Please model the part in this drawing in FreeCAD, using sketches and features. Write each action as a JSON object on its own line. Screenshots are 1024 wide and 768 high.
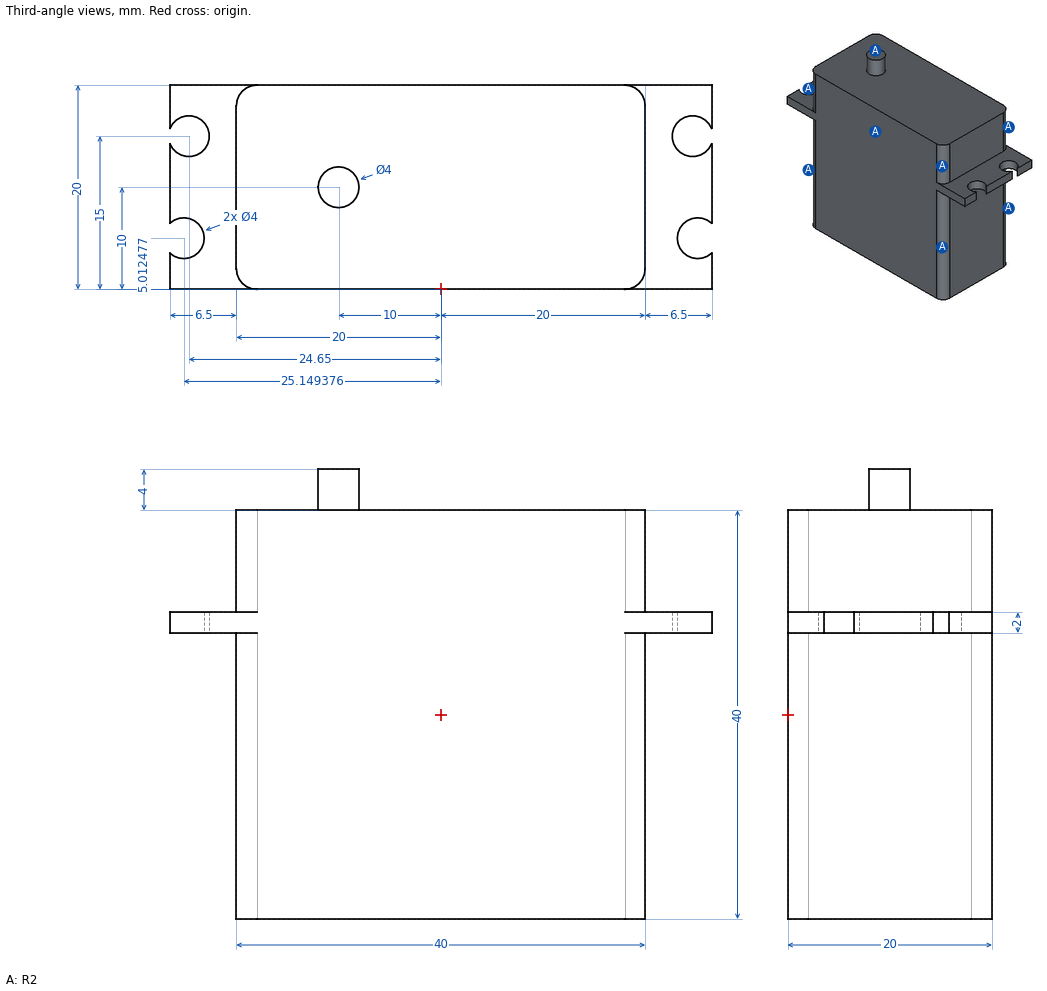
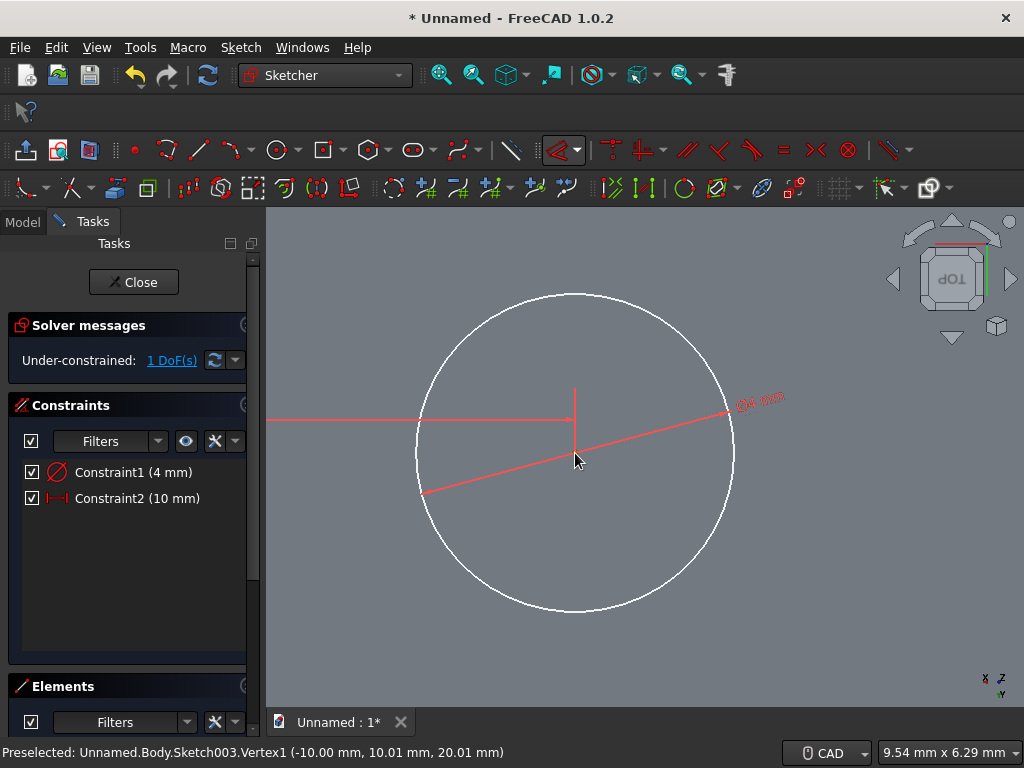
{"action": "key", "text": "i"}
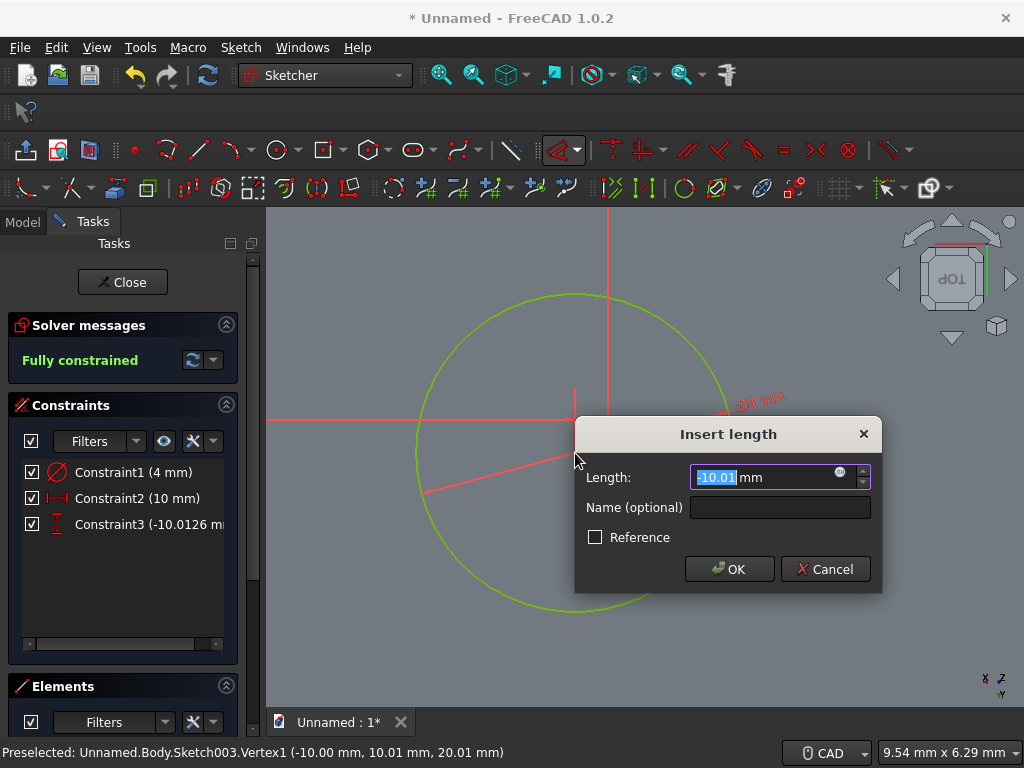
{"action": "type", "text": "-10"}
{"action": "key", "text": "Return"}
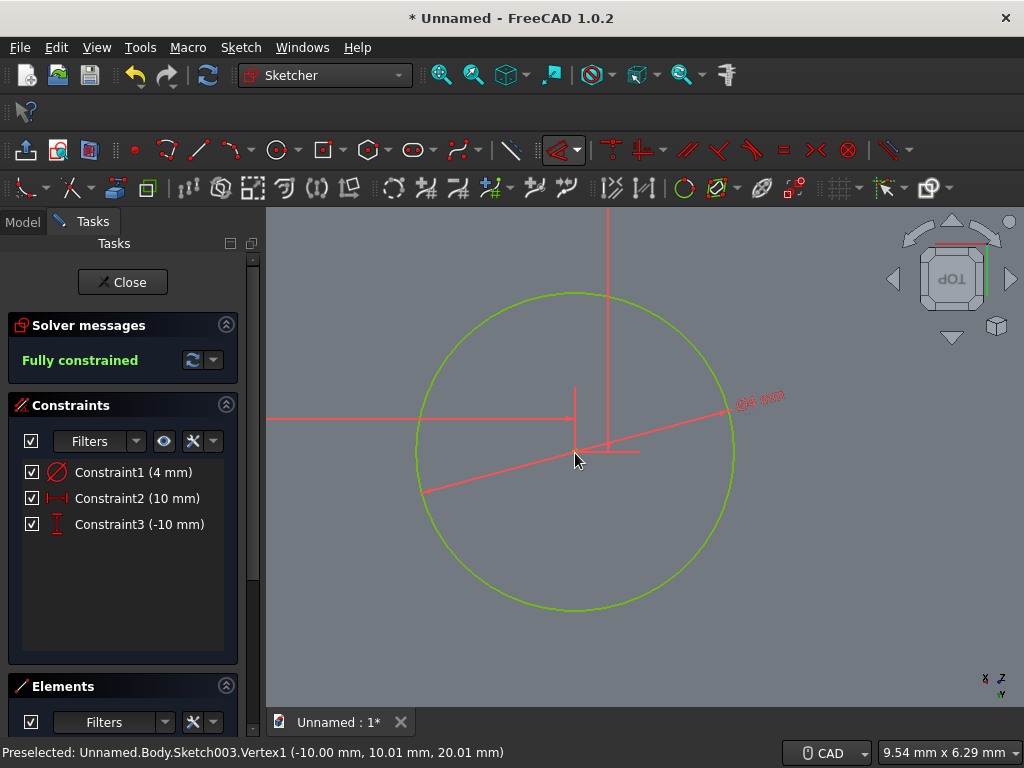
{"action": "left_click", "coordinate": [123, 282]}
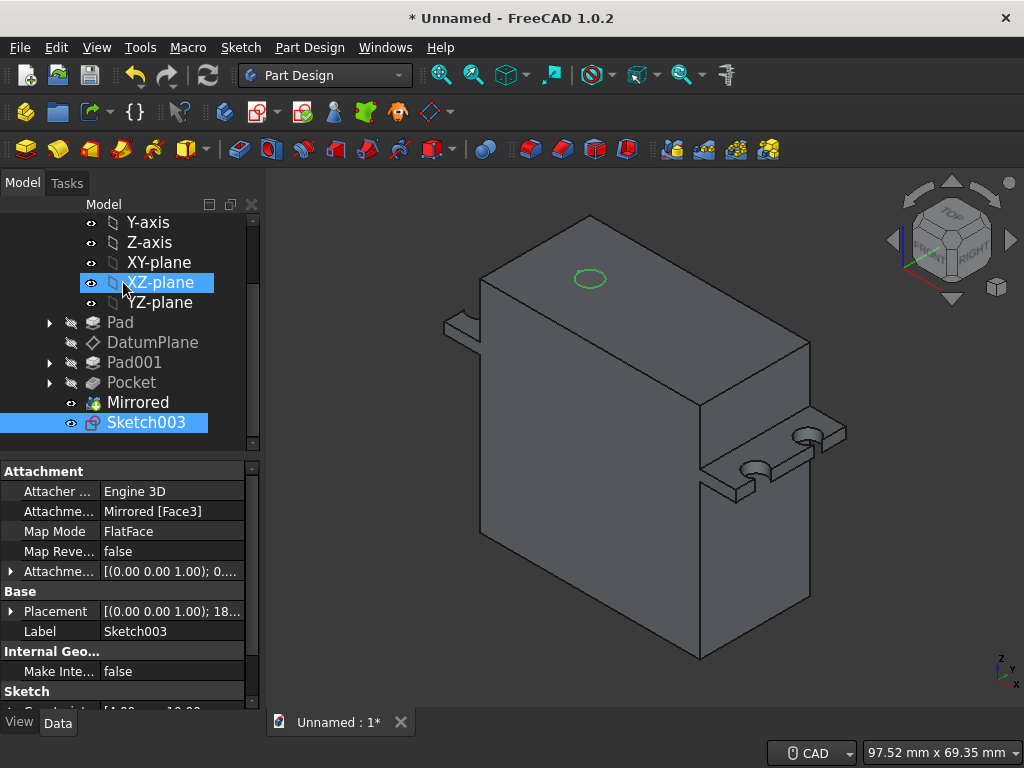
{"action": "left_click", "coordinate": [26, 150]}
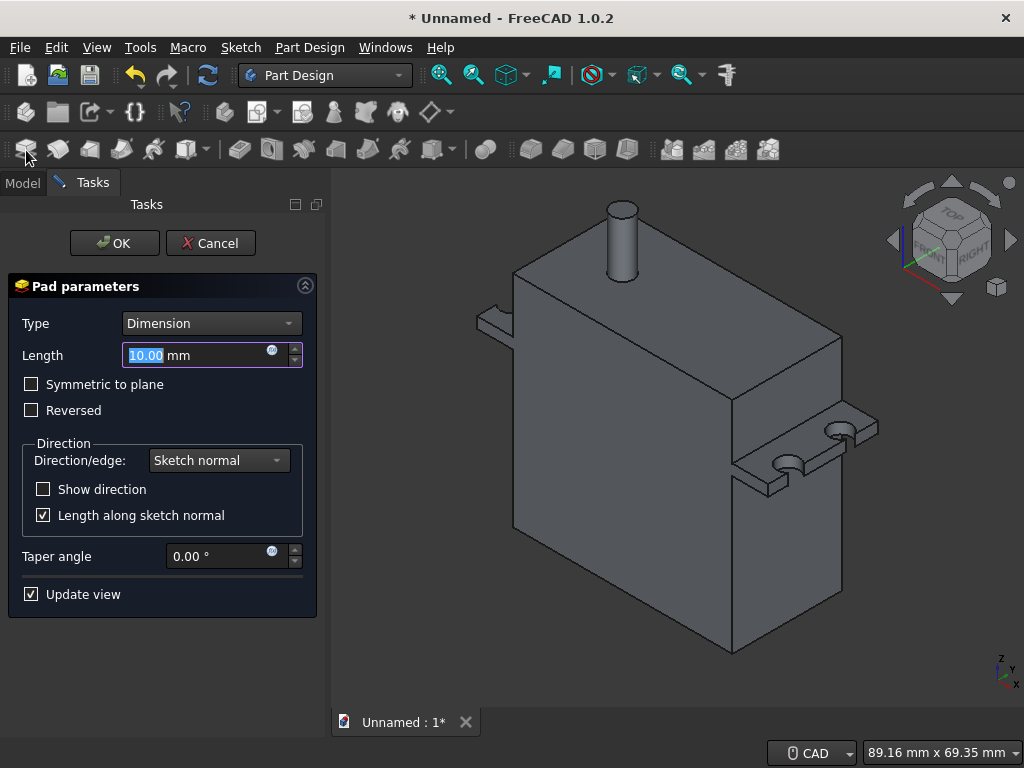
{"action": "type", "text": "4"}
{"action": "key", "text": "Tab"}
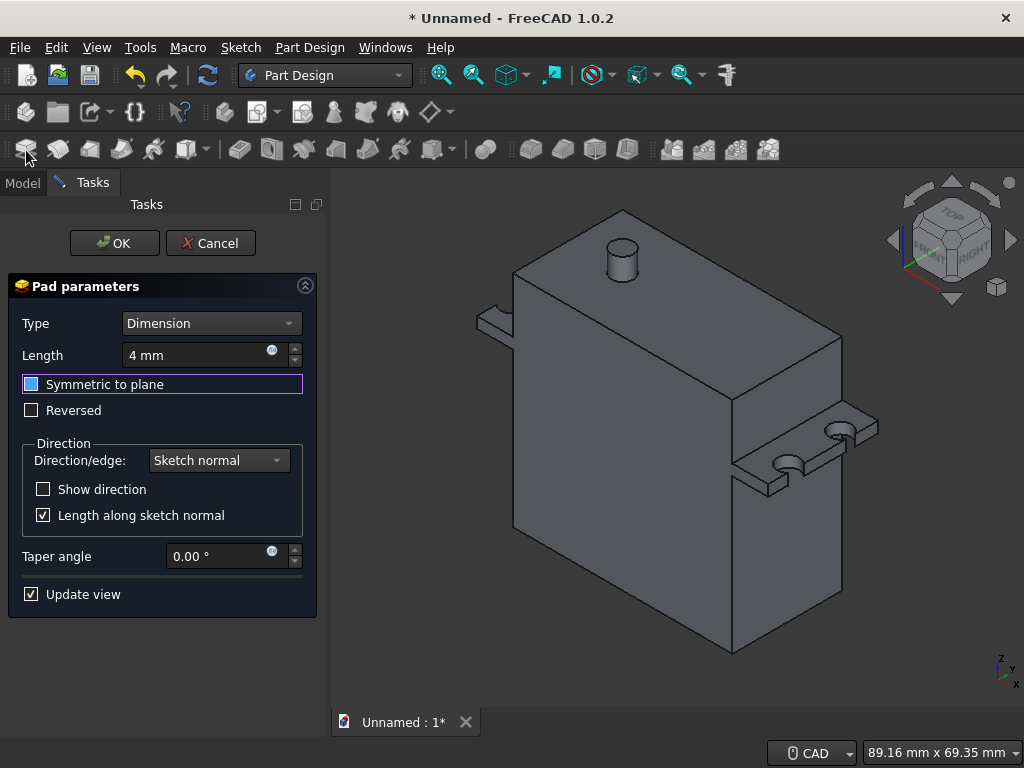
{"action": "left_click", "coordinate": [115, 243]}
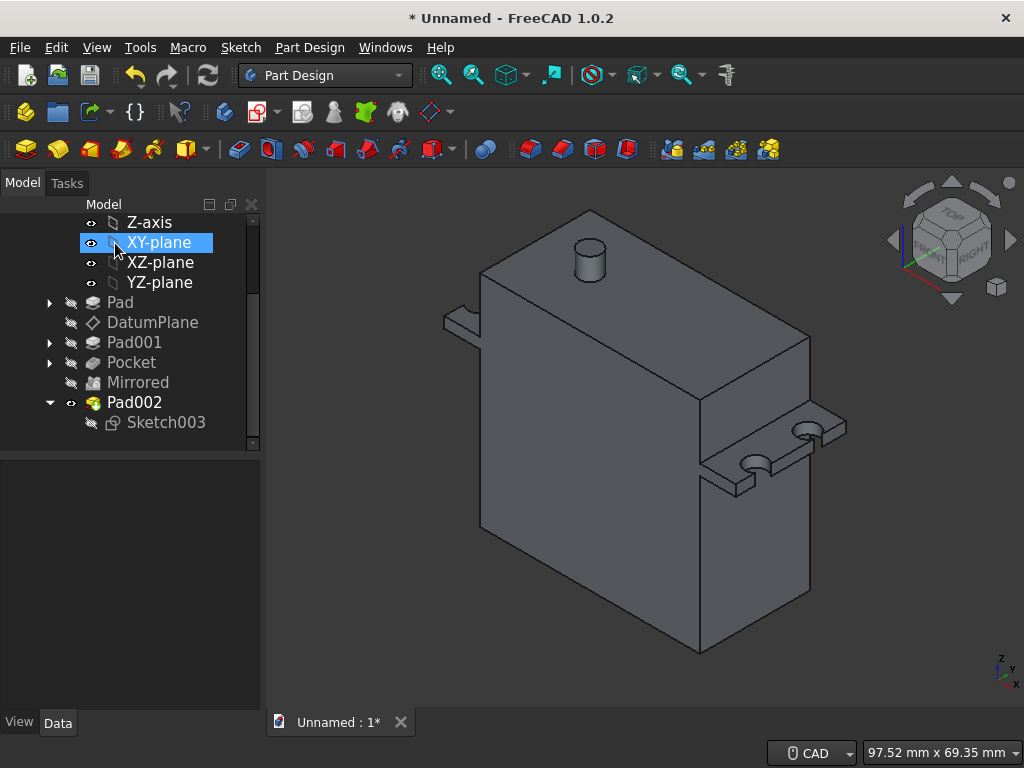
{"action": "key", "text": "v f"}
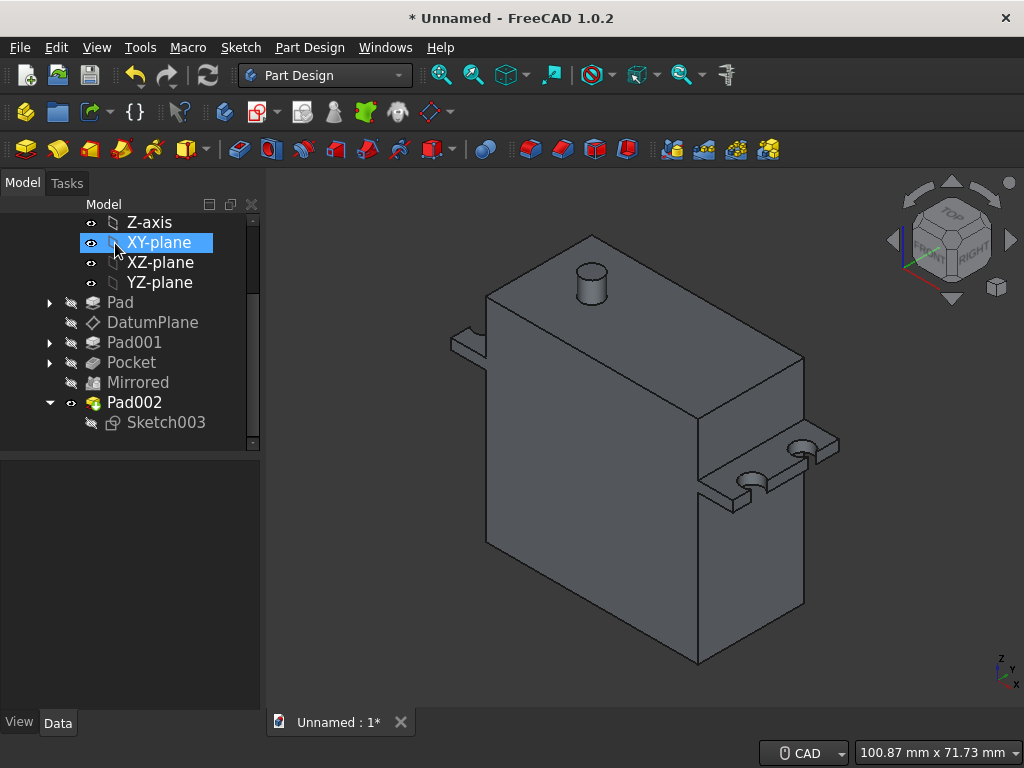
{"action": "left_click", "coordinate": [698, 578]}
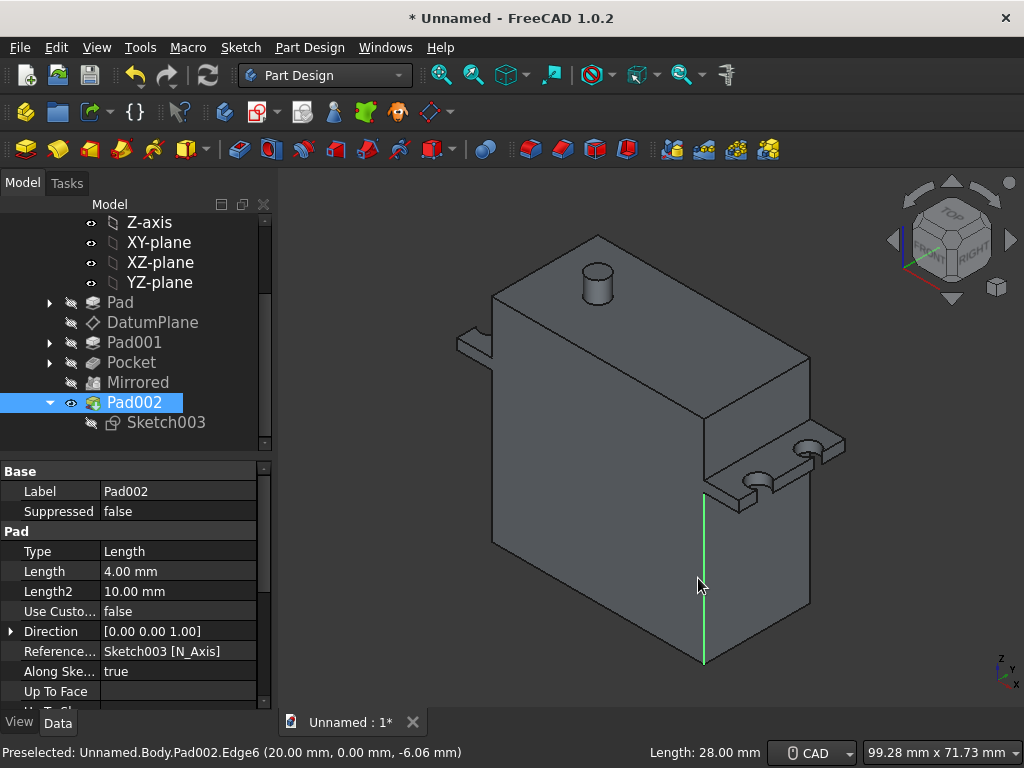
{"action": "left_click", "coordinate": [704, 449], "text": "ctrl"}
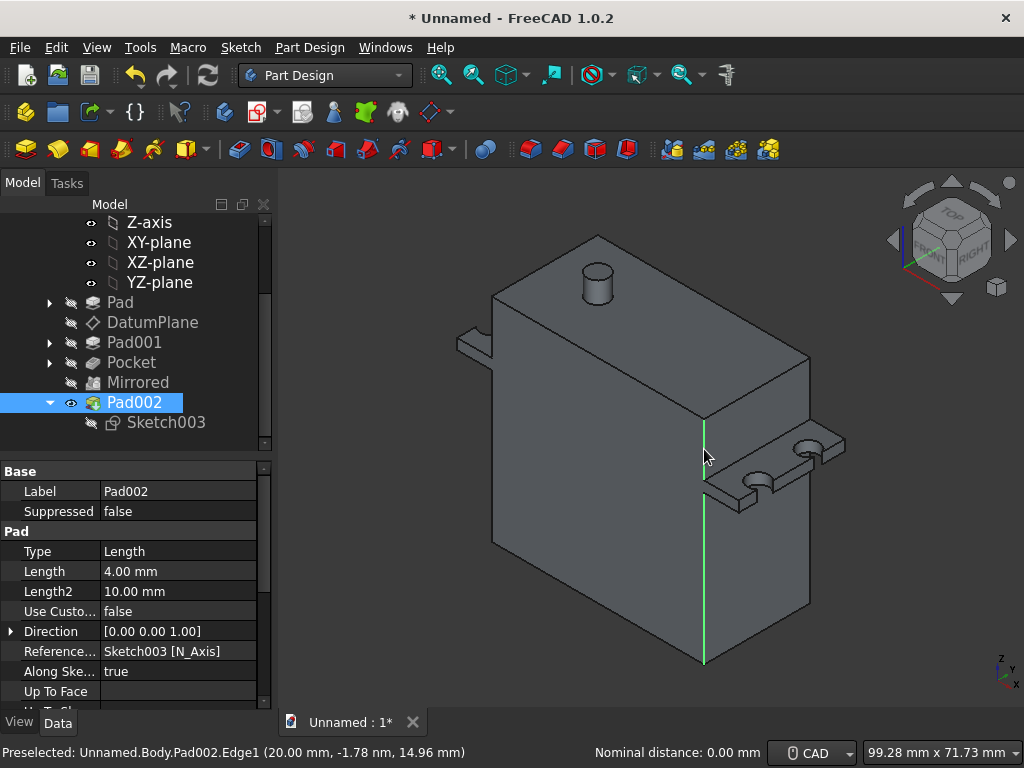
{"action": "key", "text": "2"}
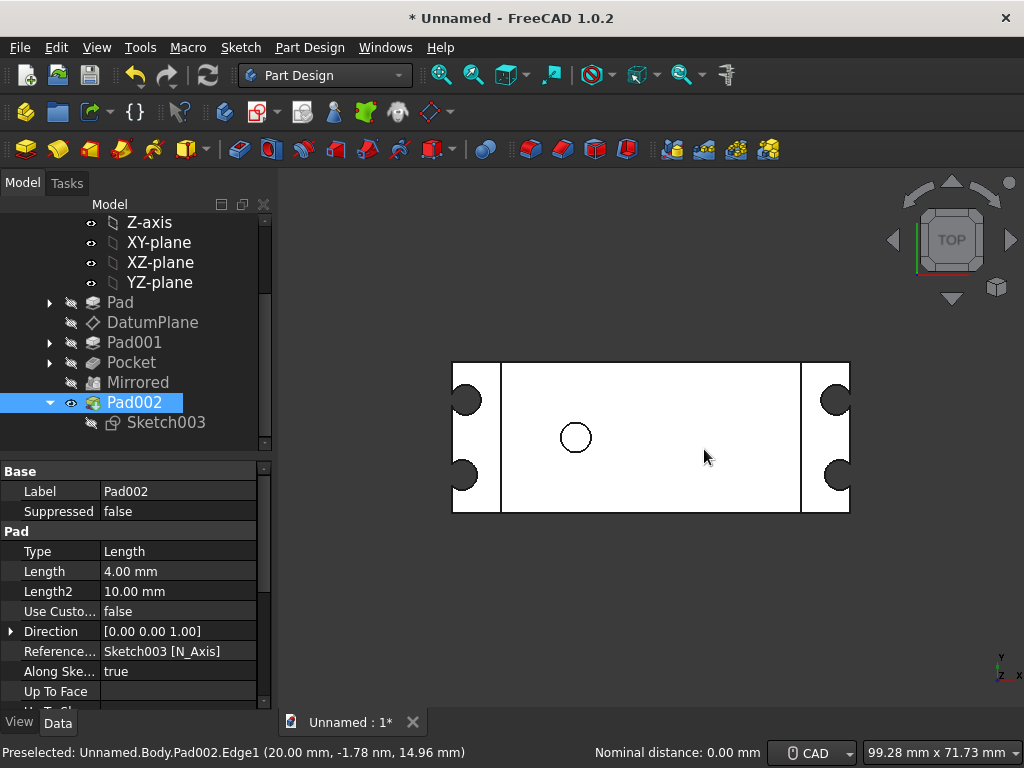
{"action": "key", "text": "0"}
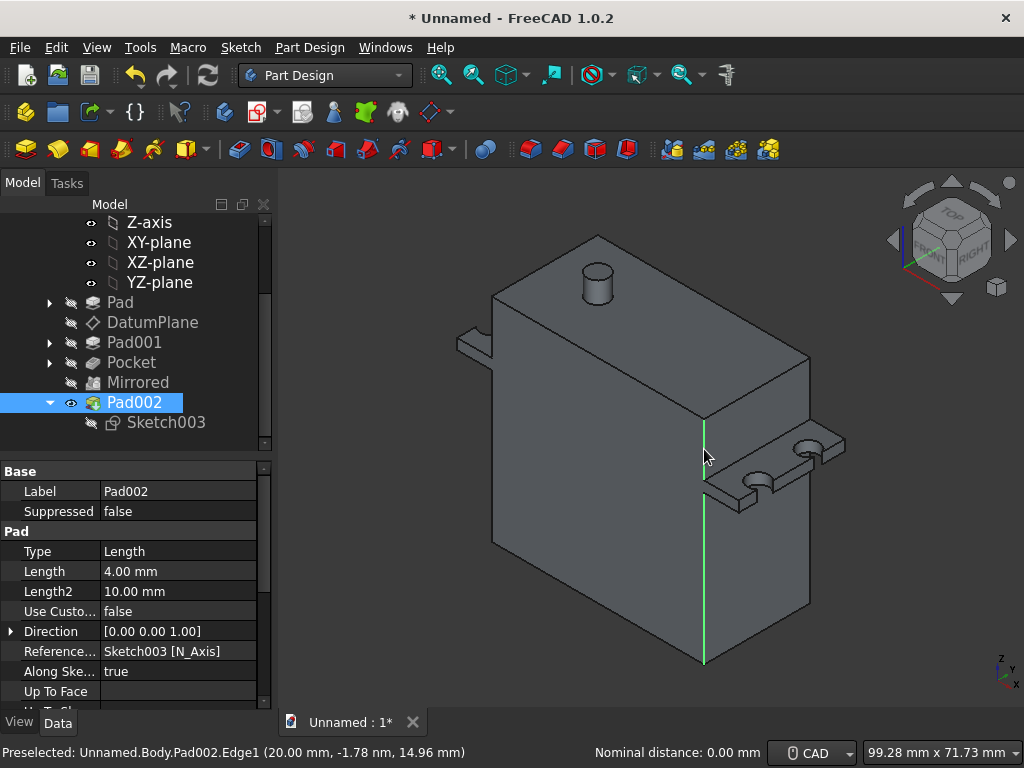
{"action": "key", "text": "1"}